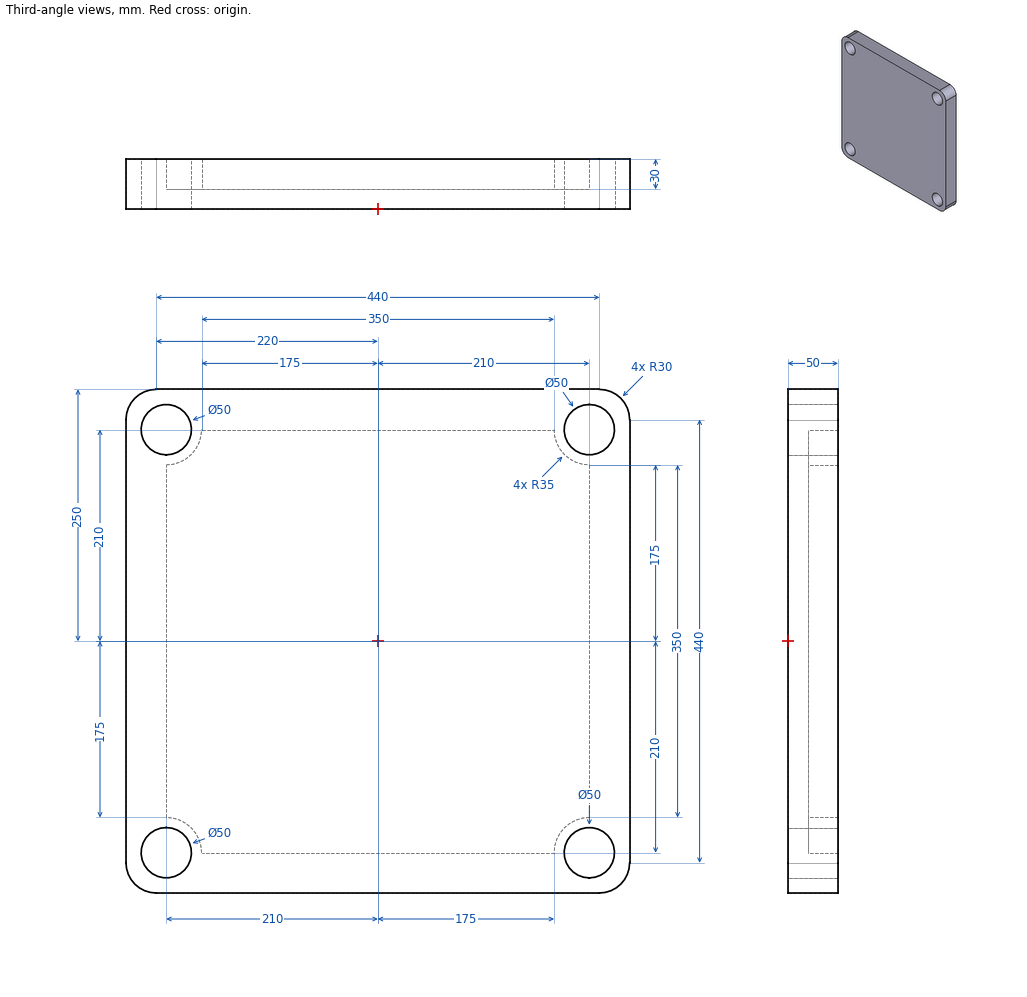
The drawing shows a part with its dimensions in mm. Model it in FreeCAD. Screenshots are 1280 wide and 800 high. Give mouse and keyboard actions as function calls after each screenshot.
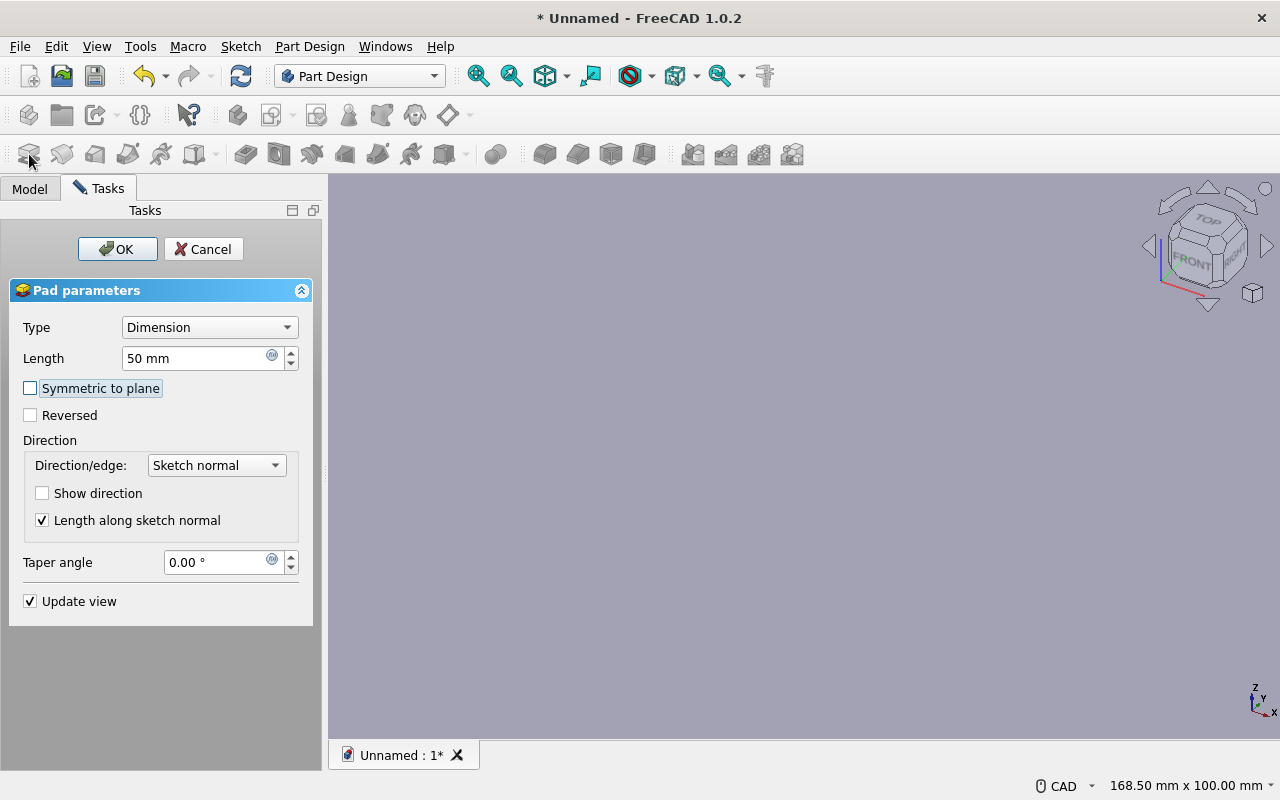
click(31, 415)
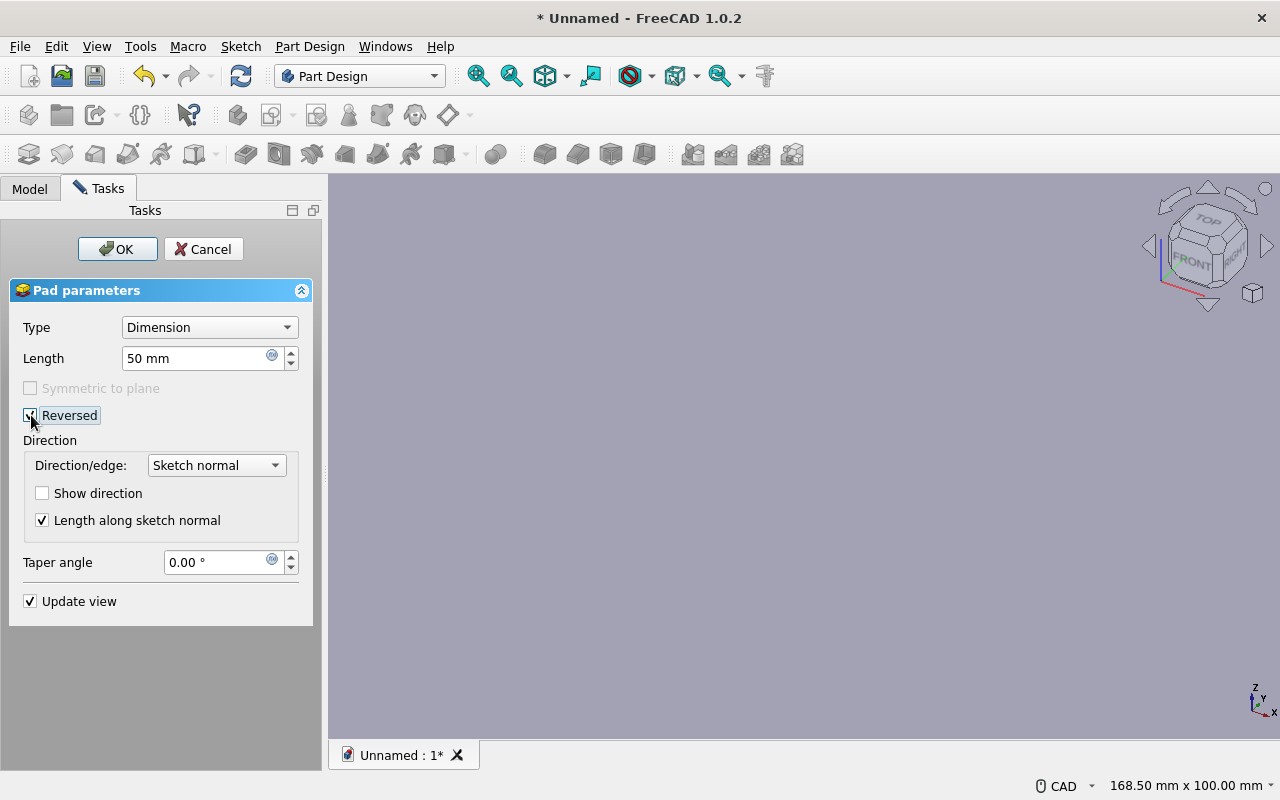
click(118, 249)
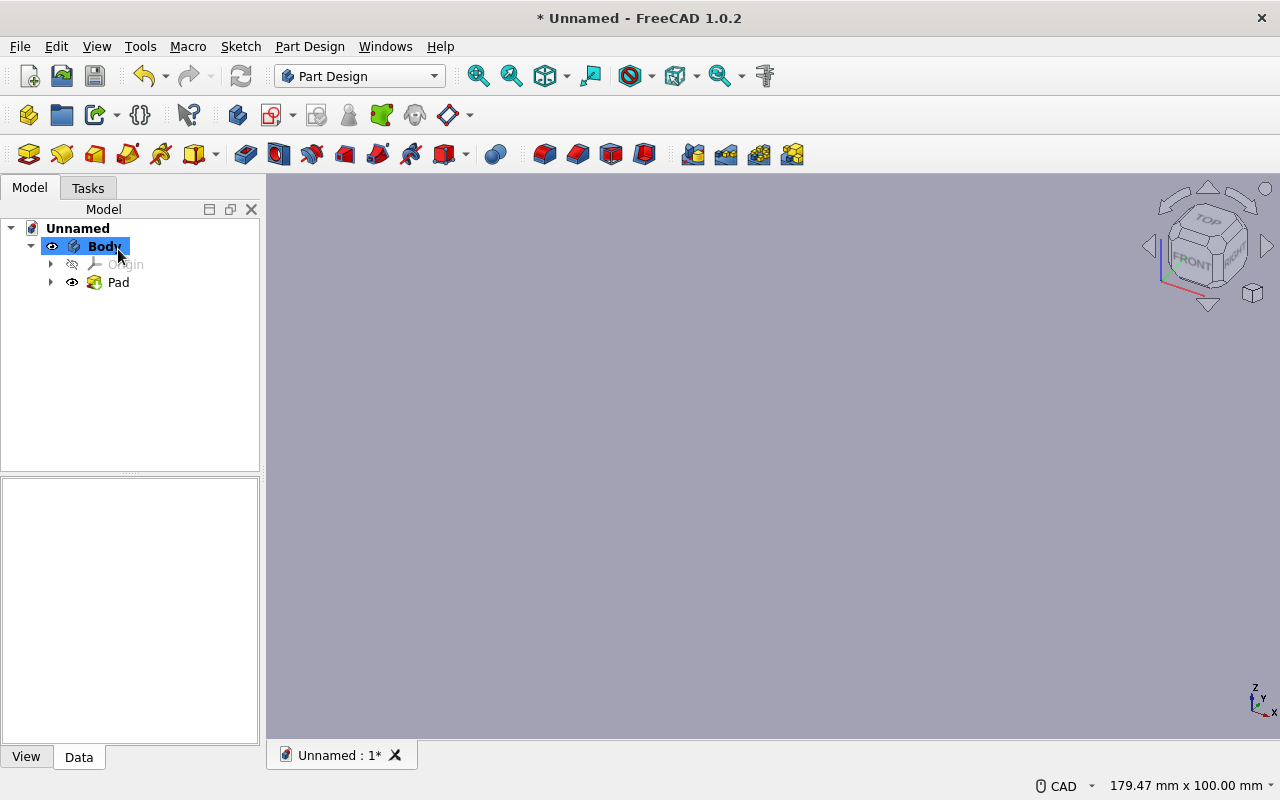
click(479, 76)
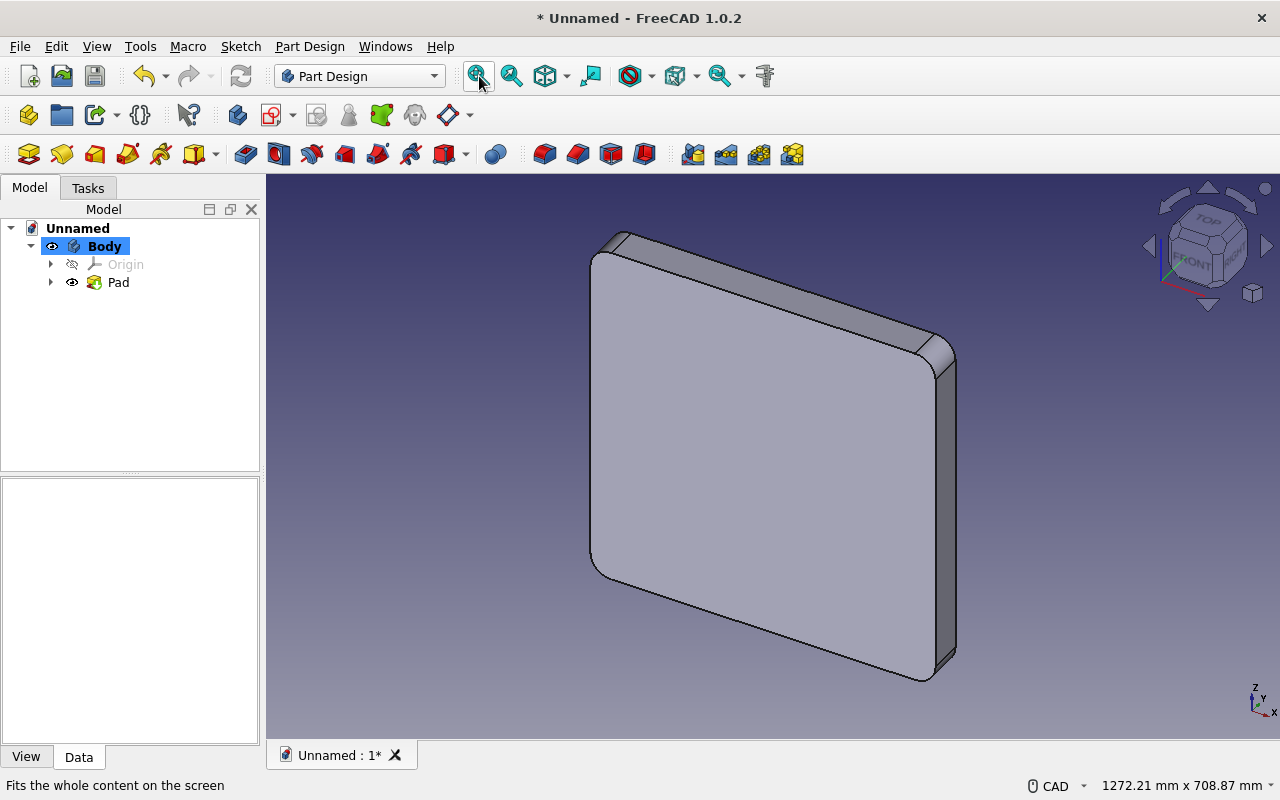
key(4)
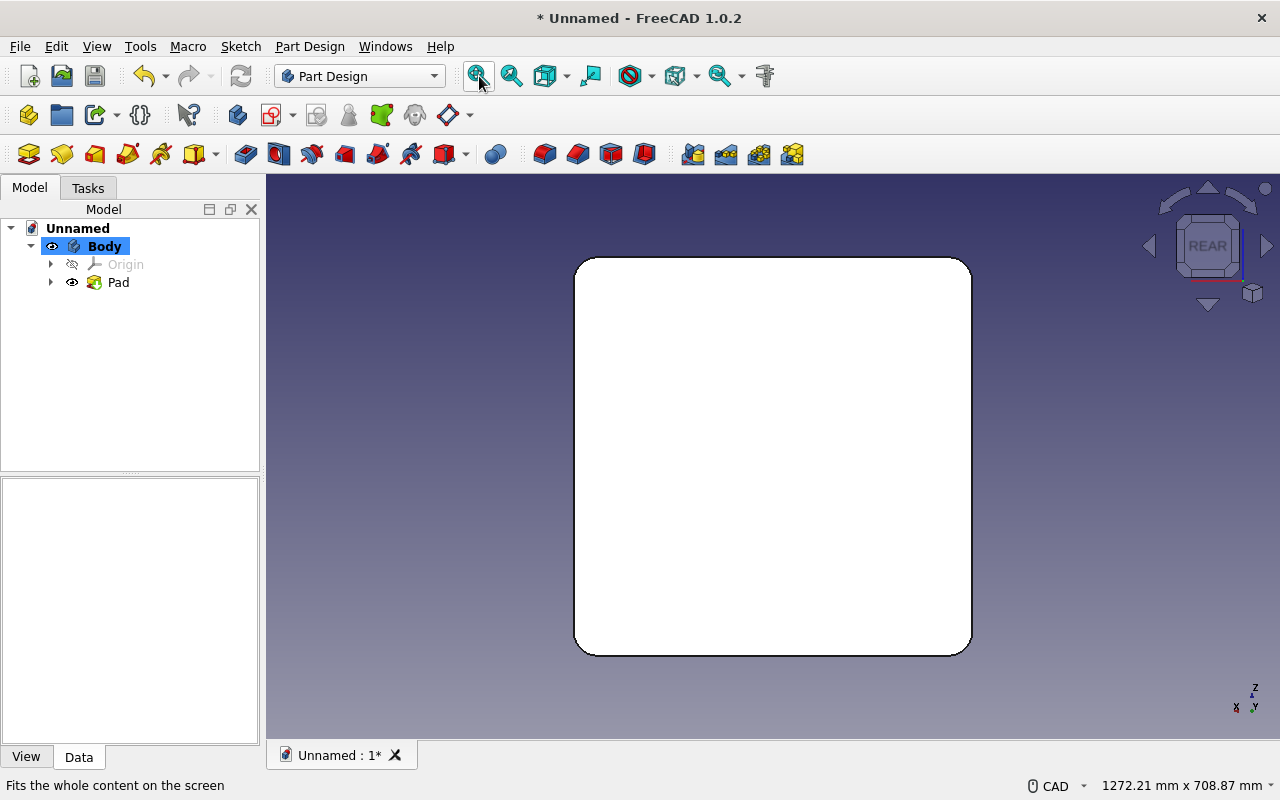
click(773, 456)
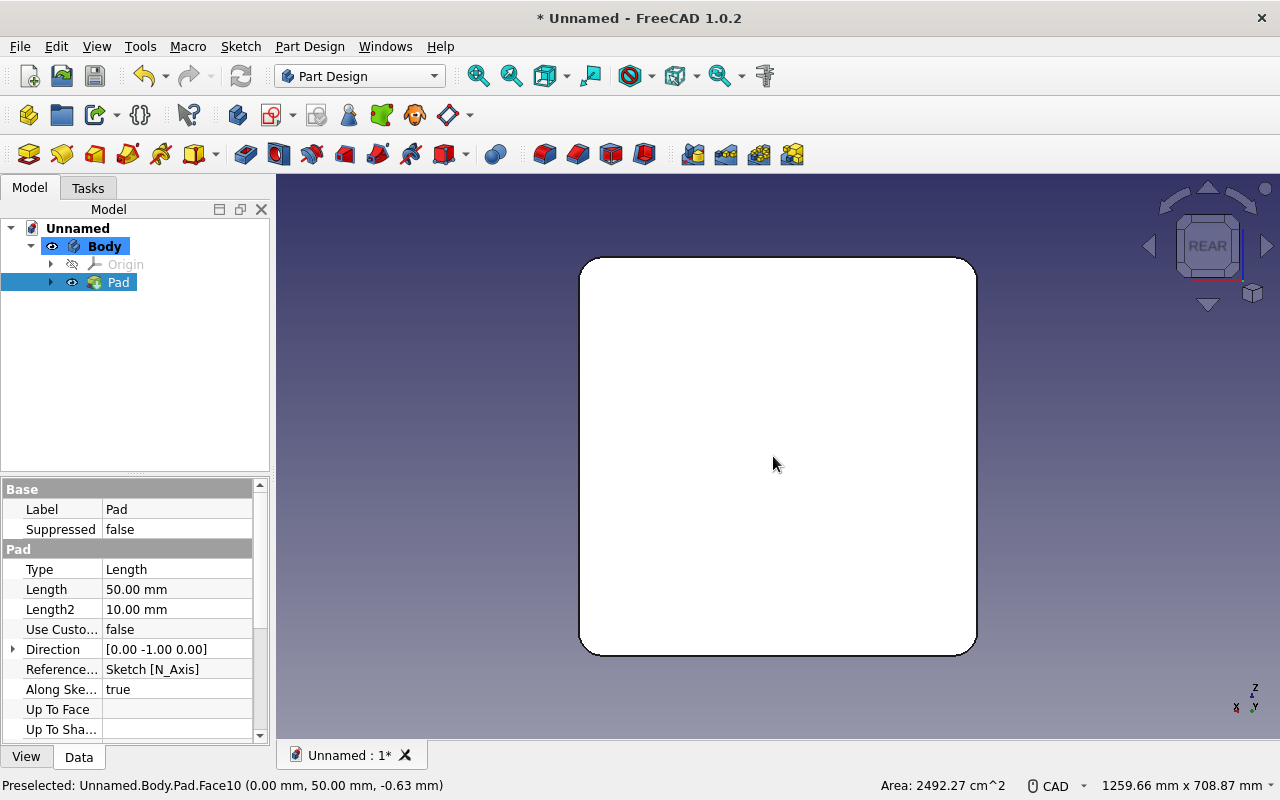
click(270, 116)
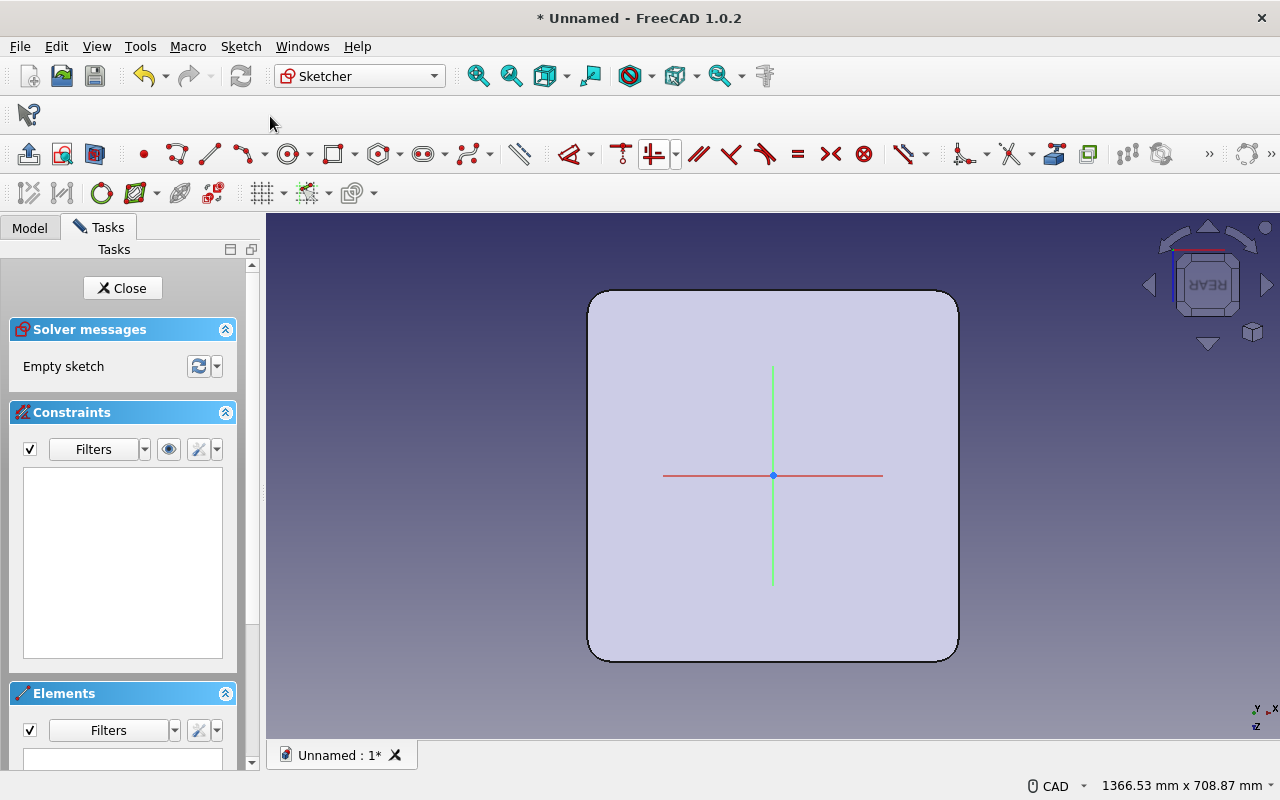
click(210, 154)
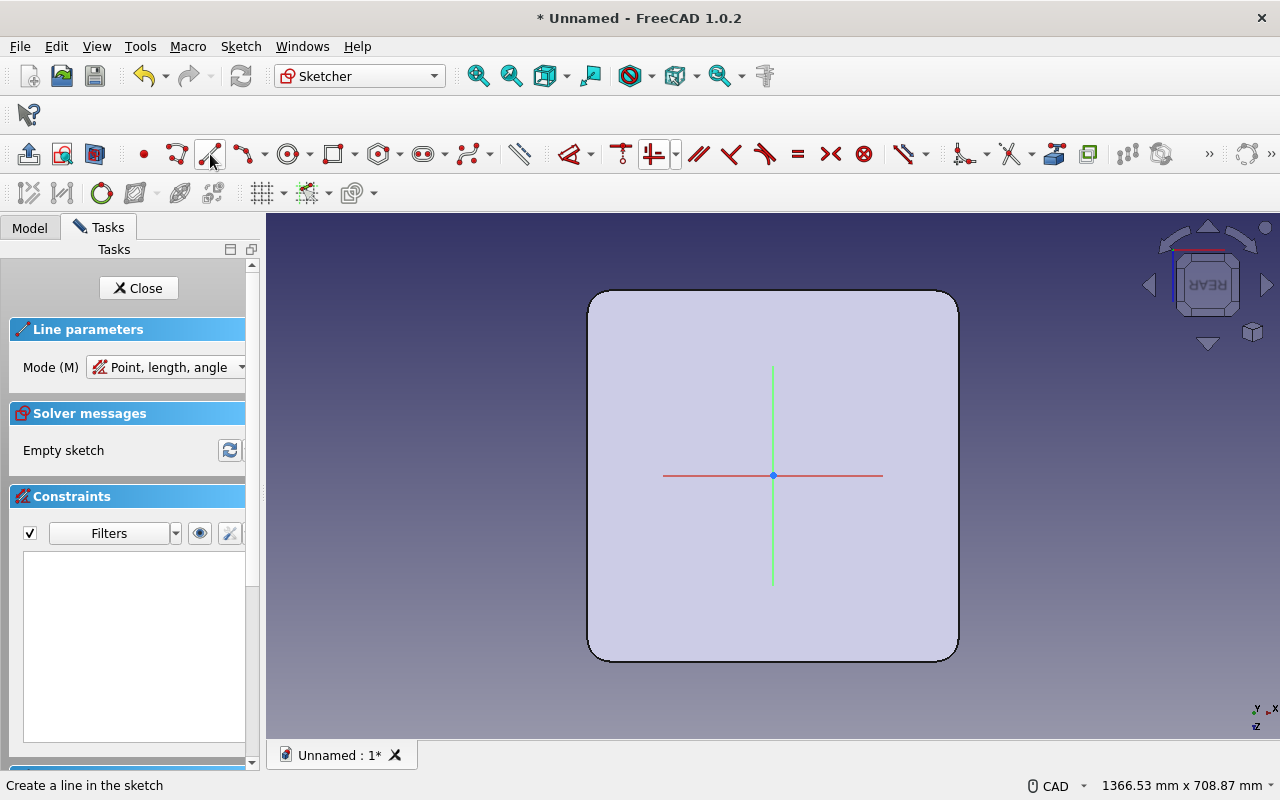
click(643, 632)
click(903, 632)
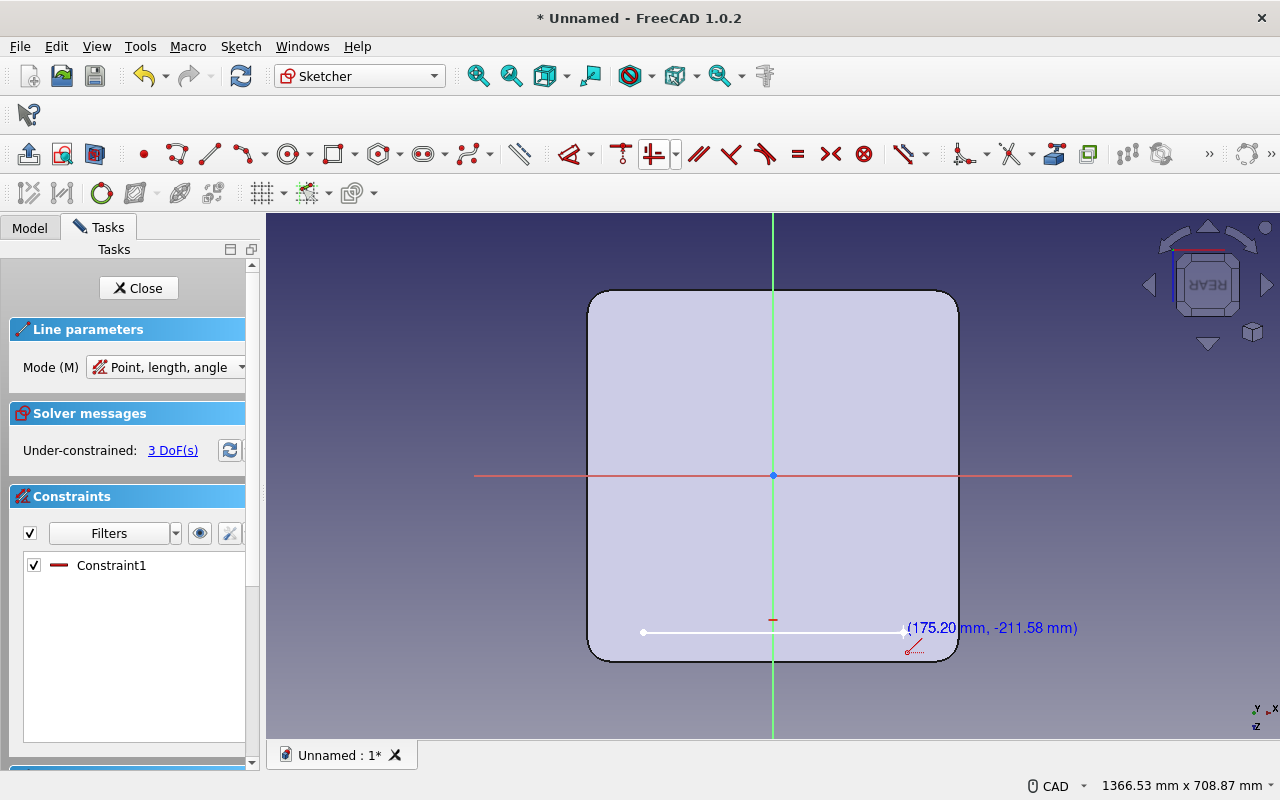
click(929, 606)
click(929, 346)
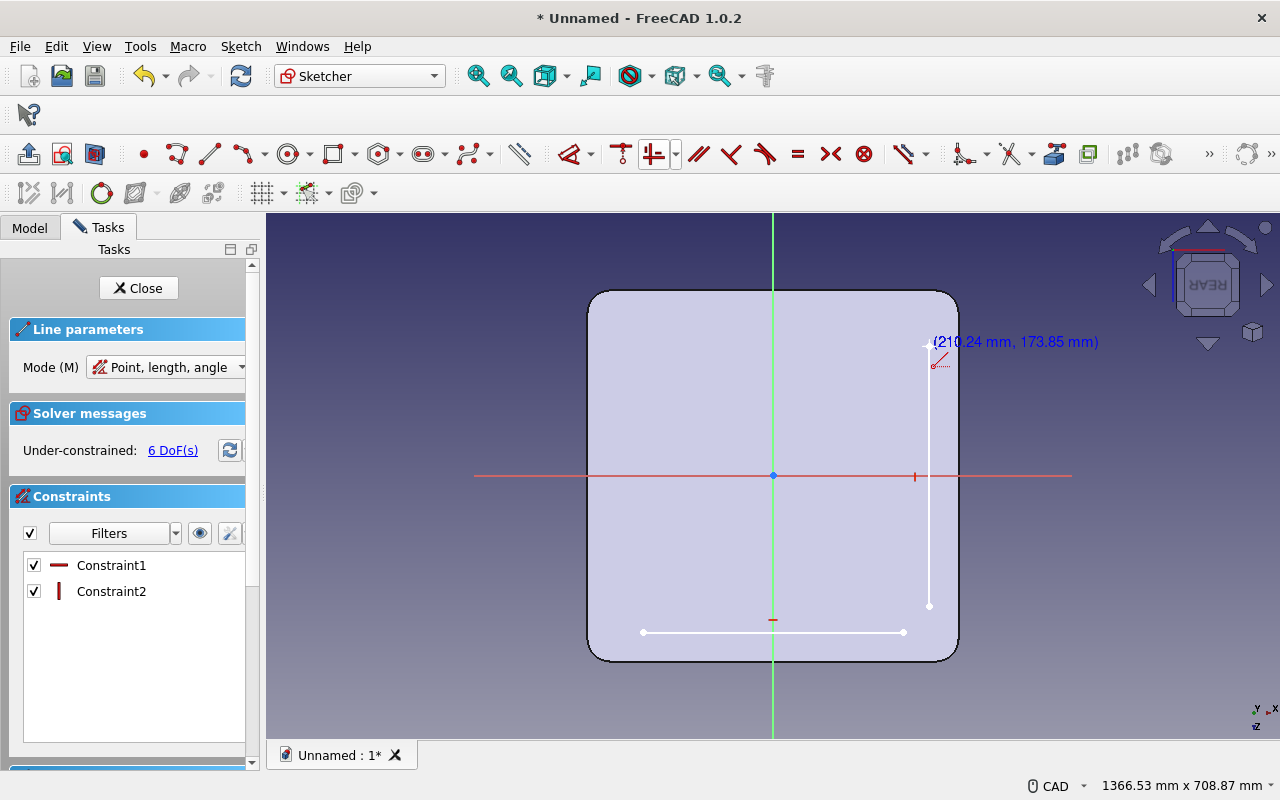
click(903, 320)
click(643, 320)